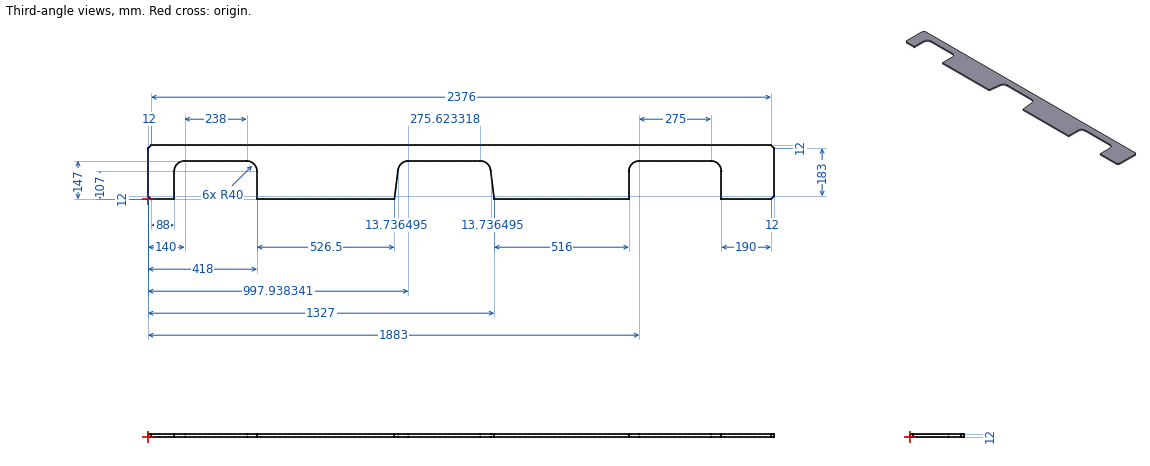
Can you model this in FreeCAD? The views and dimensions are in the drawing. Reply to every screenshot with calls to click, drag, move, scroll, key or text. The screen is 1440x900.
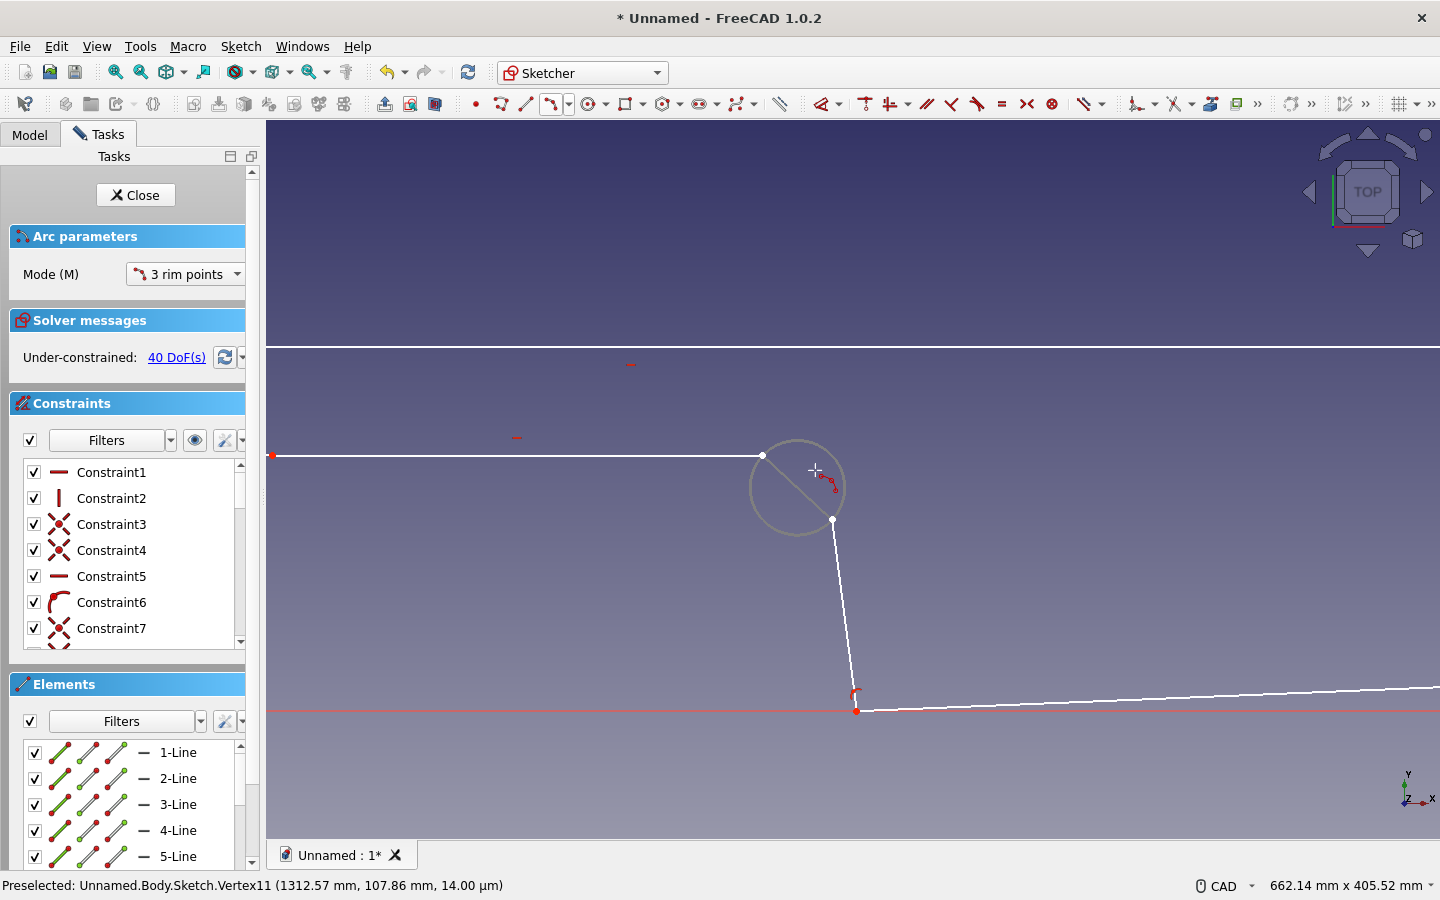
click(810, 468)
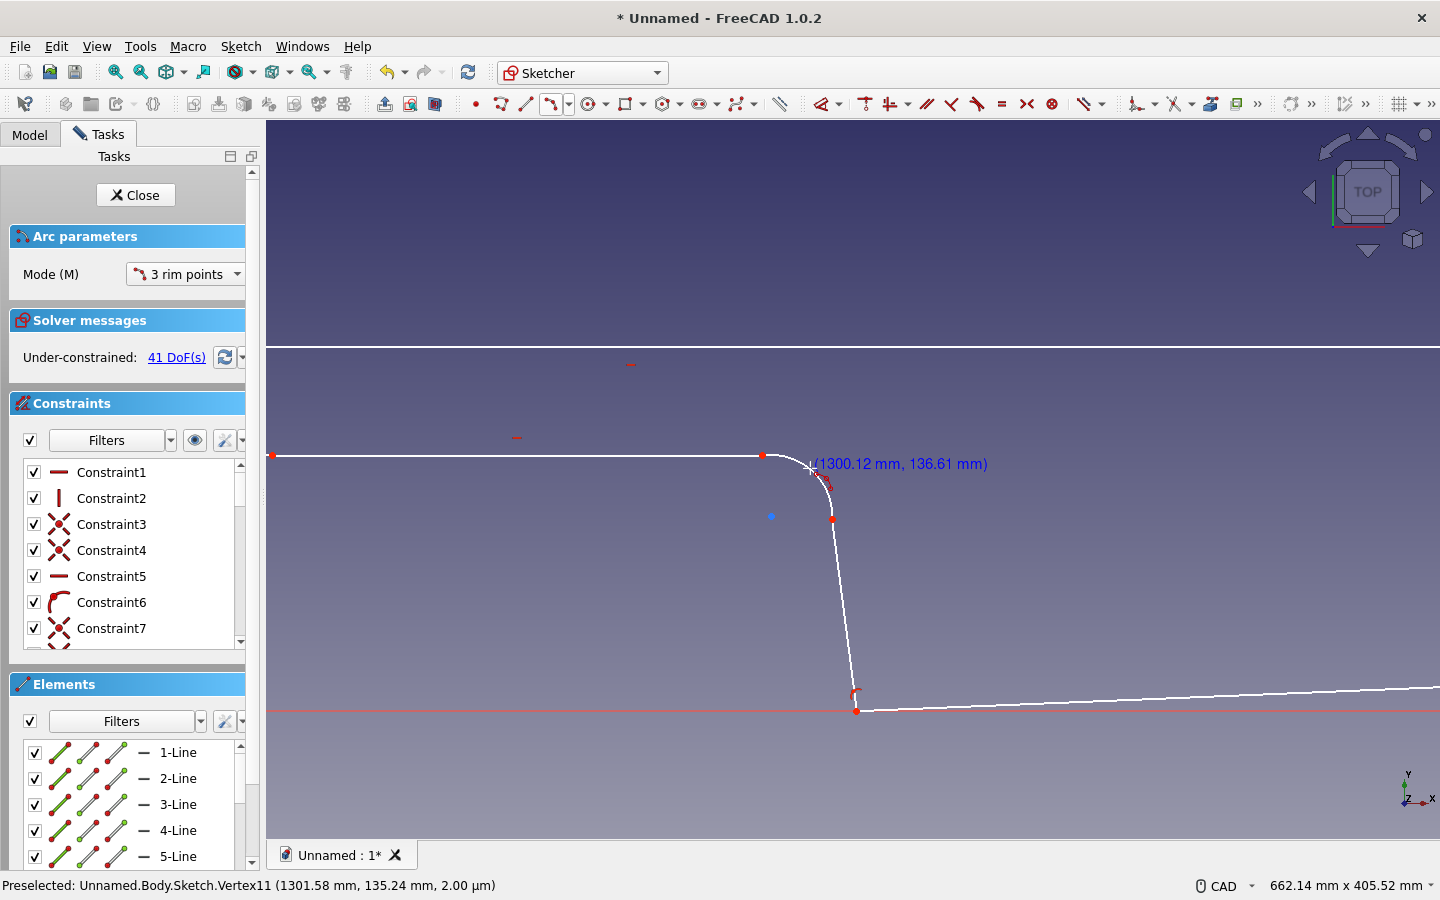
scroll(815, 470, down, 9)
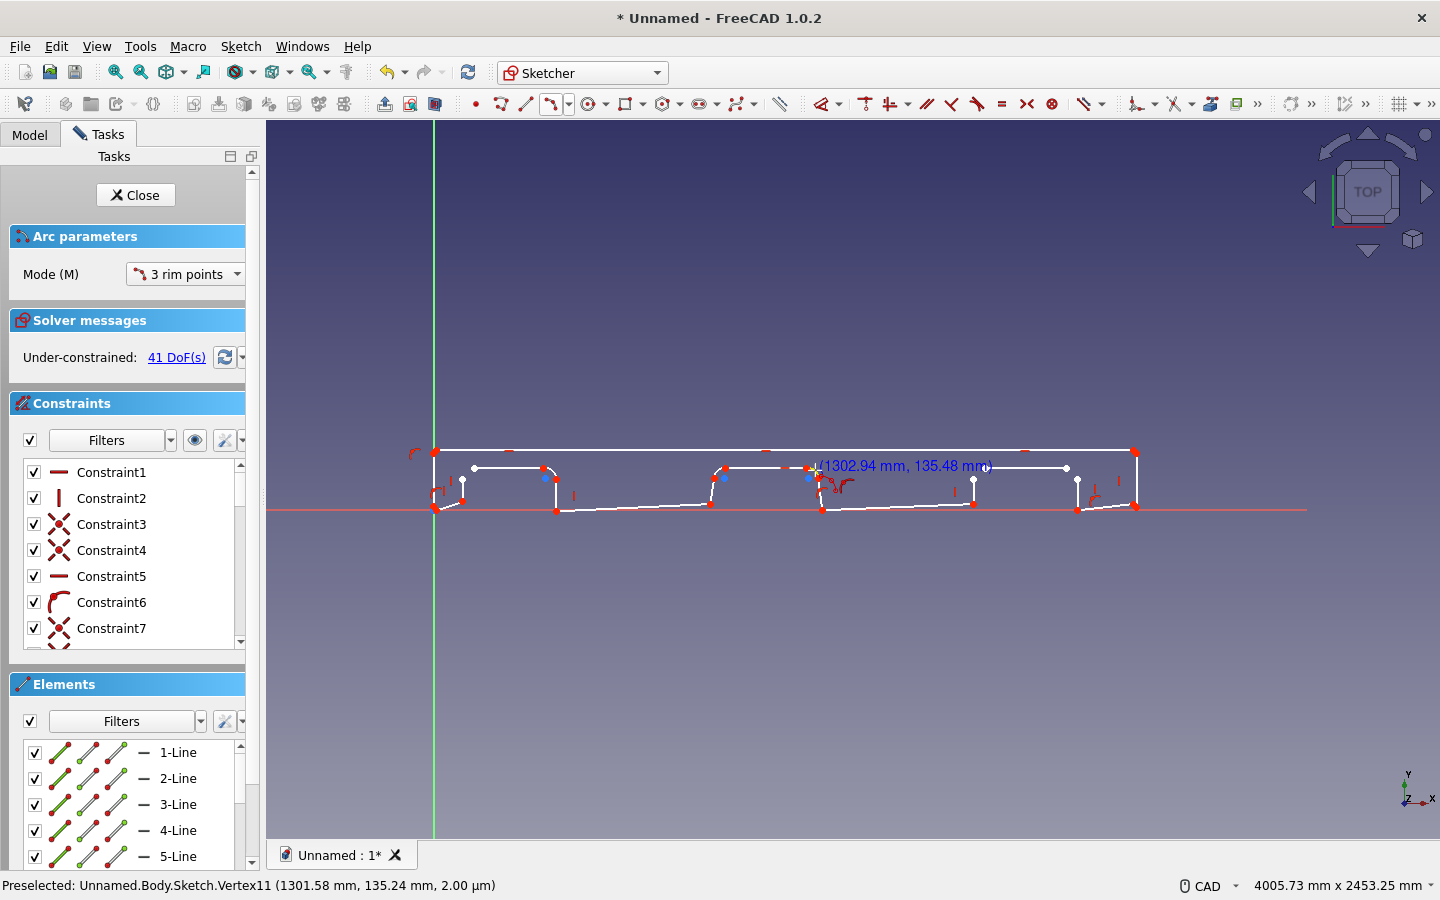
click(974, 479)
click(985, 468)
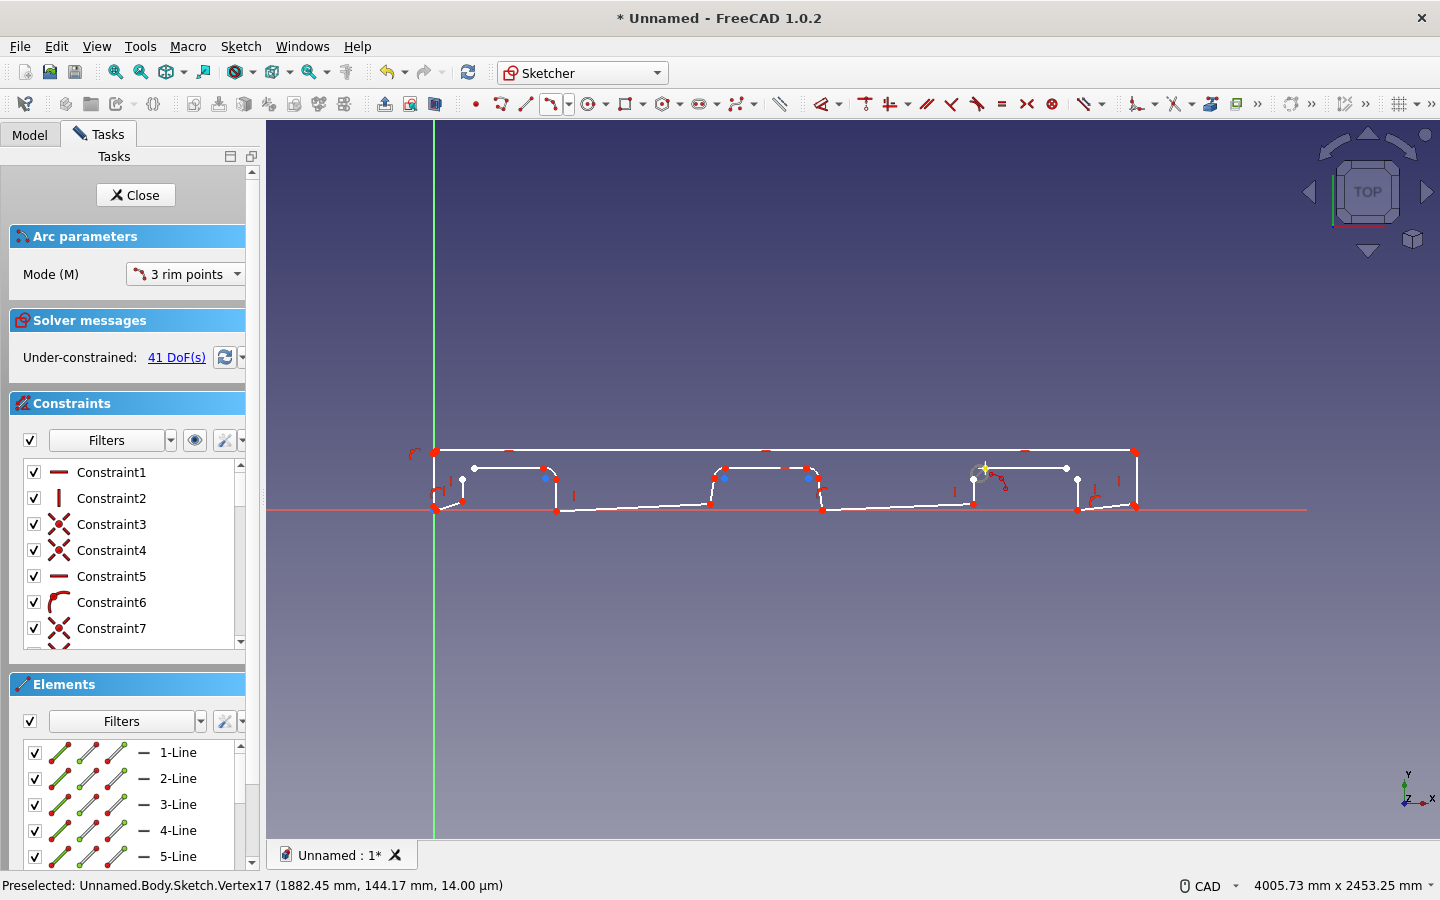
scroll(977, 471, up, 8)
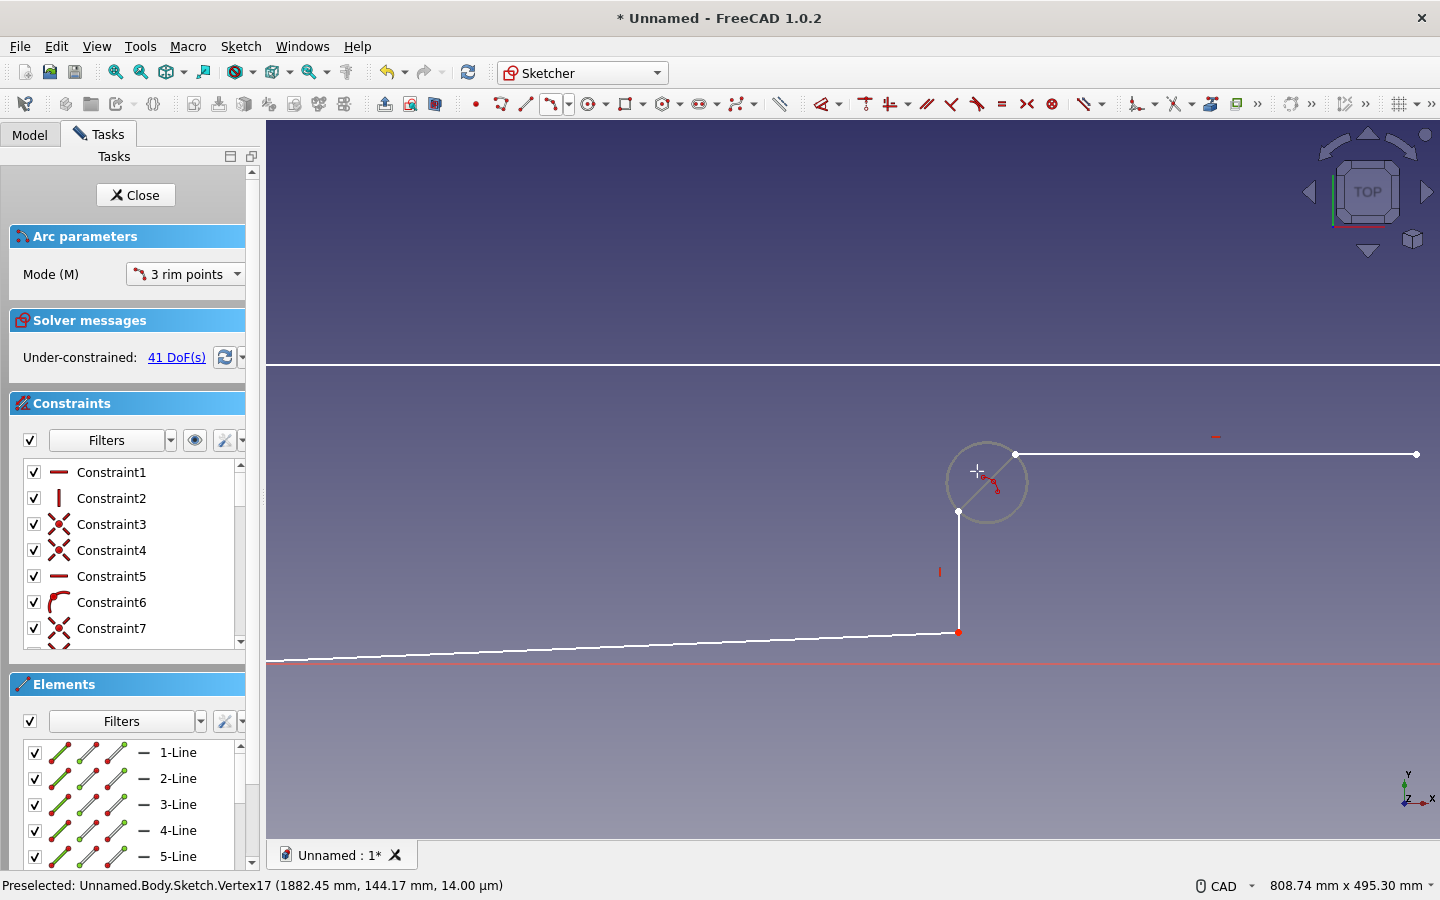
click(975, 467)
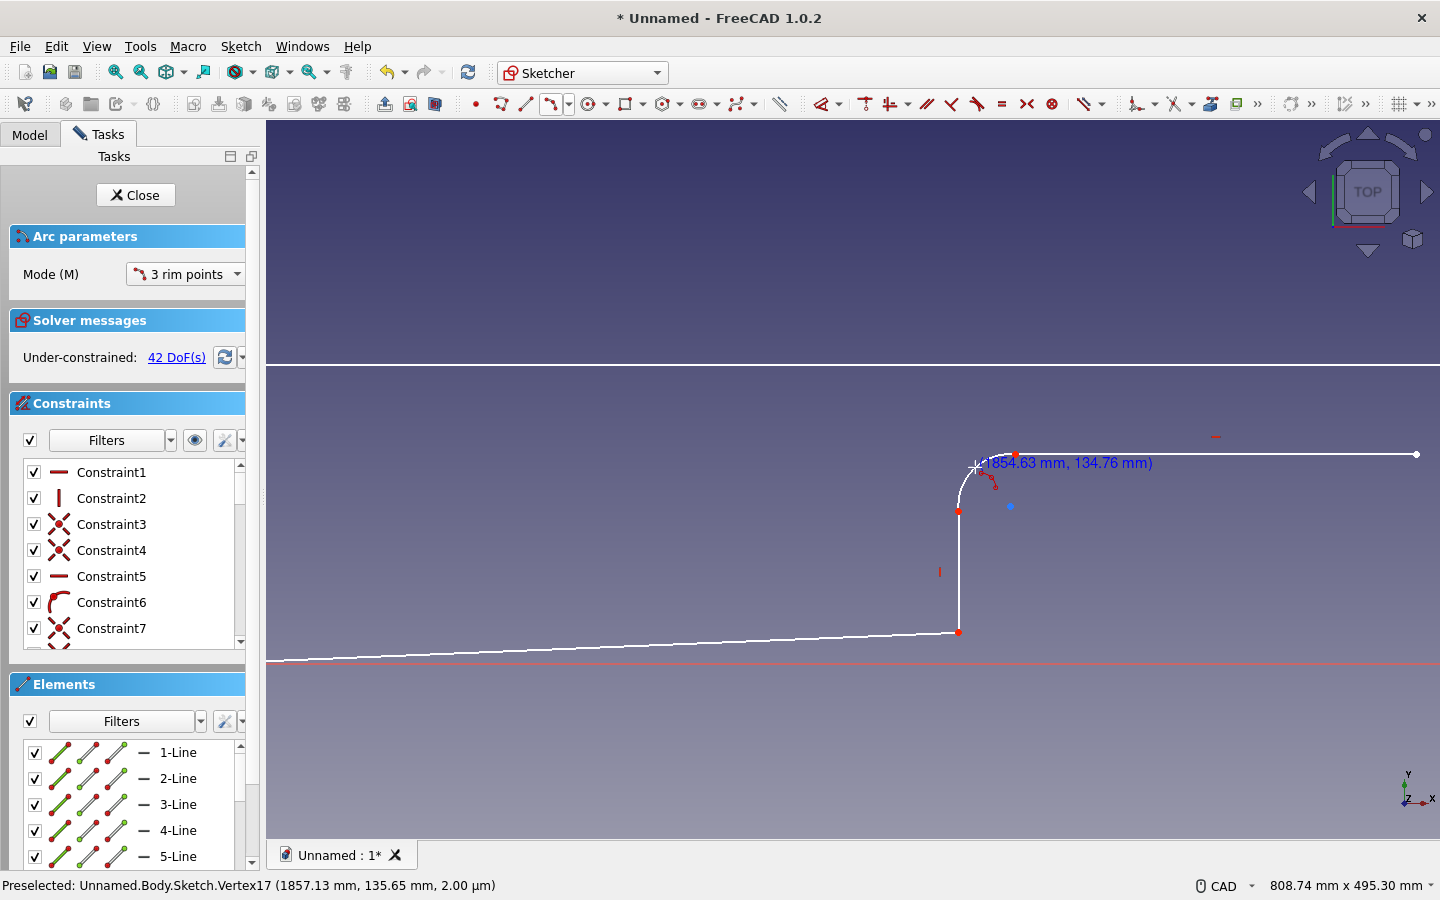
scroll(977, 471, down, 8)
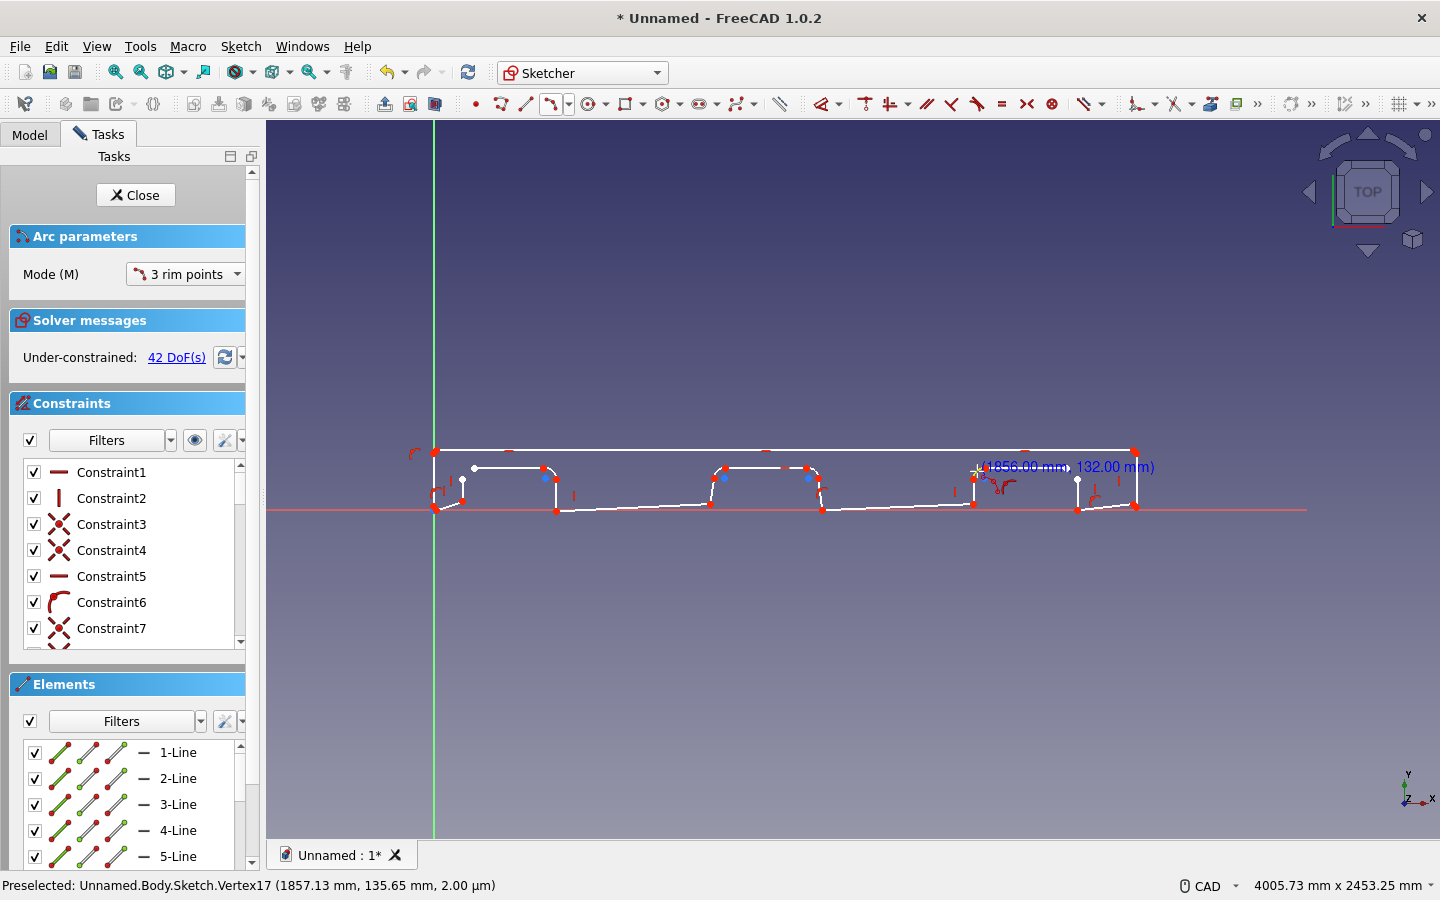
click(1066, 468)
click(1078, 479)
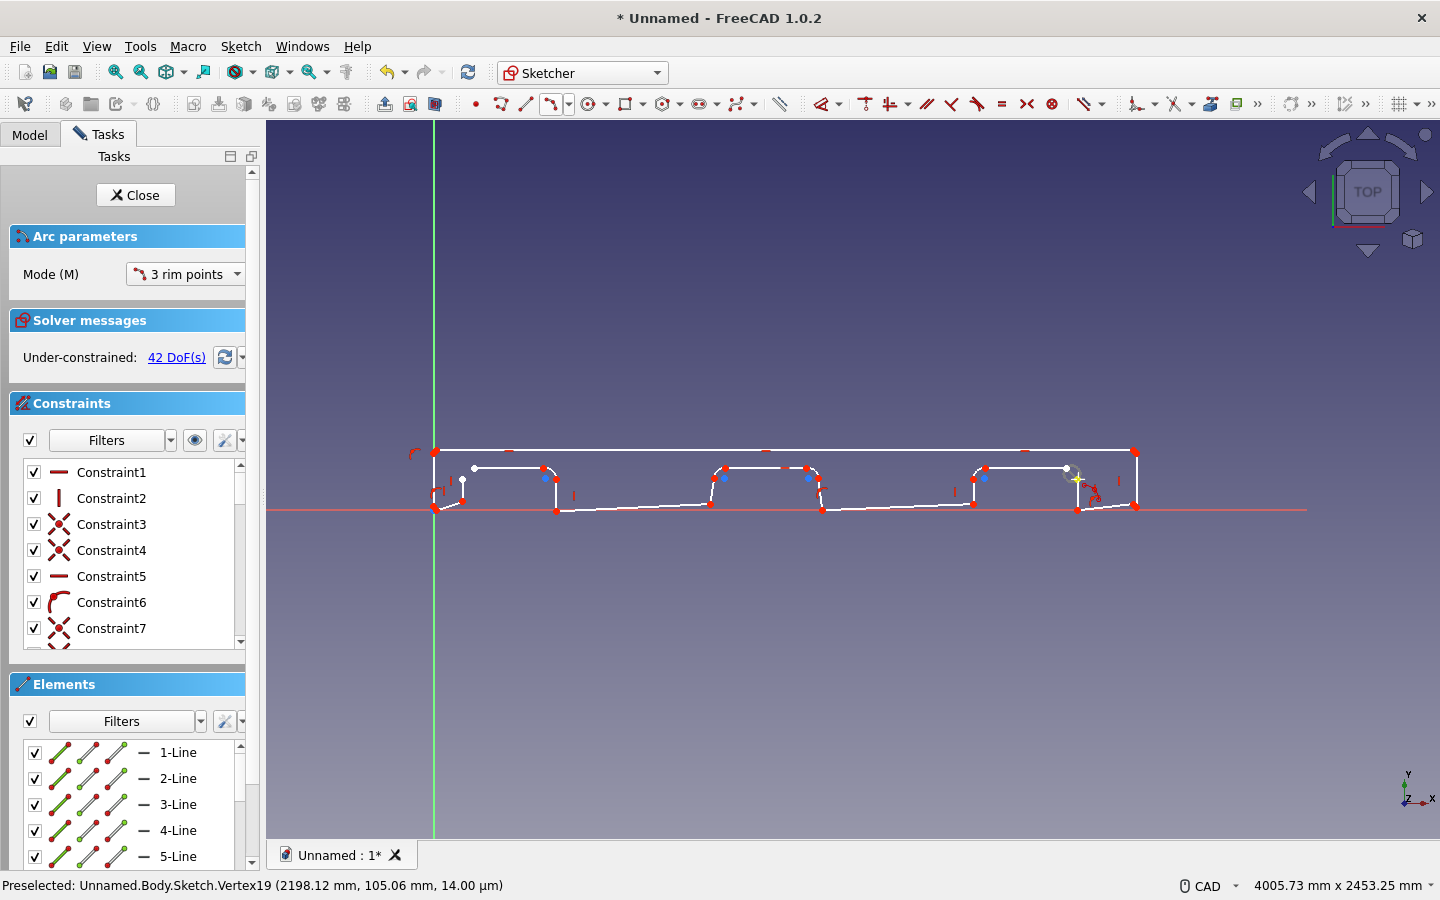
scroll(1074, 471, up, 8)